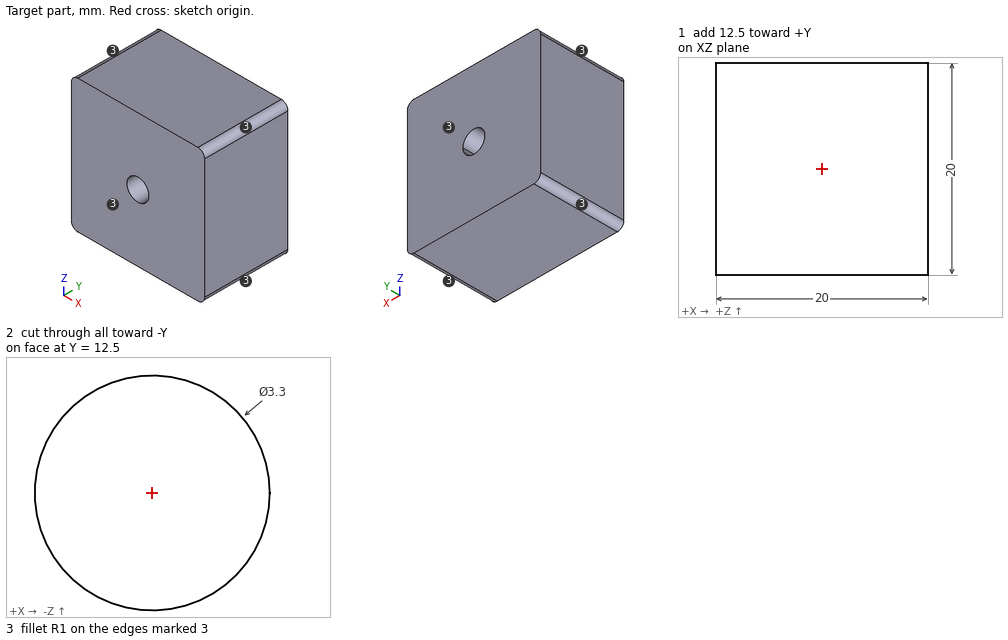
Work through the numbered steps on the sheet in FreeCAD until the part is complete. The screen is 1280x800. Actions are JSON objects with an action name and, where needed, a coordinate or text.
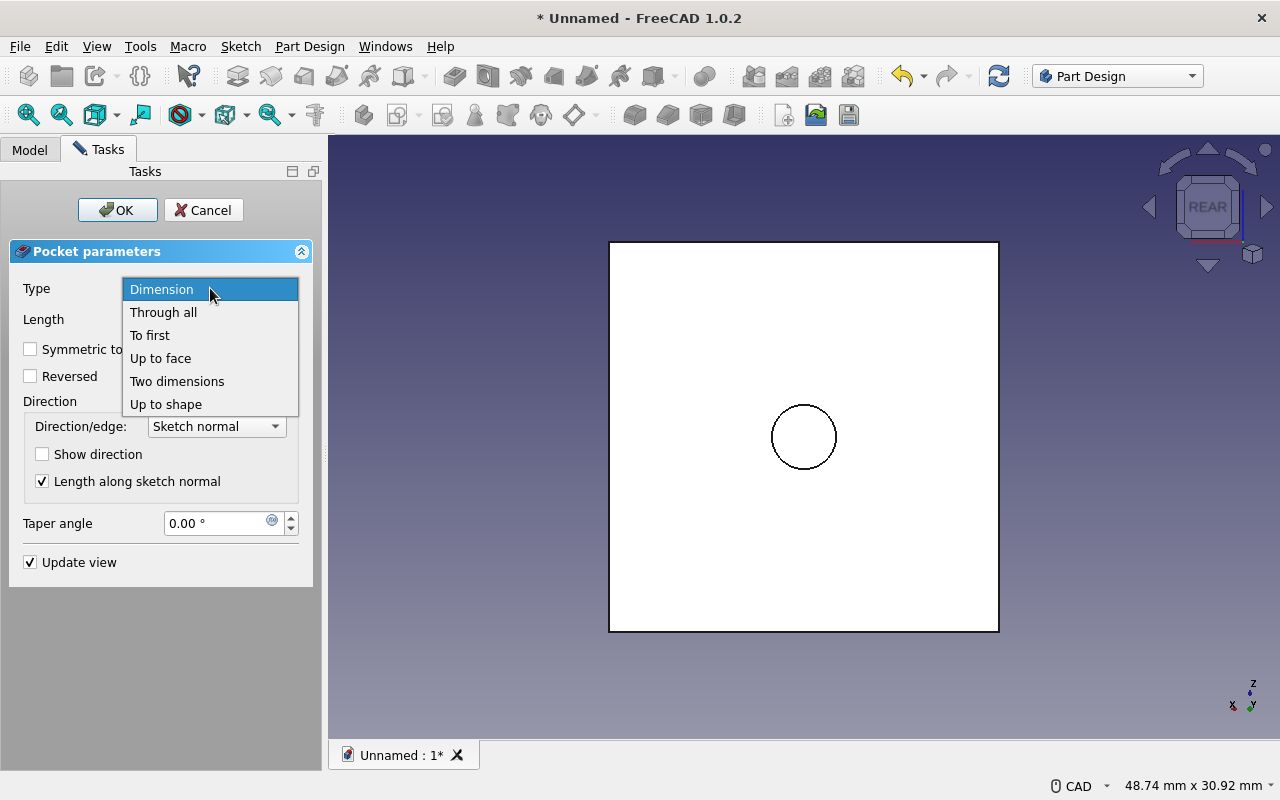
{"action": "left_click", "coordinate": [208, 312]}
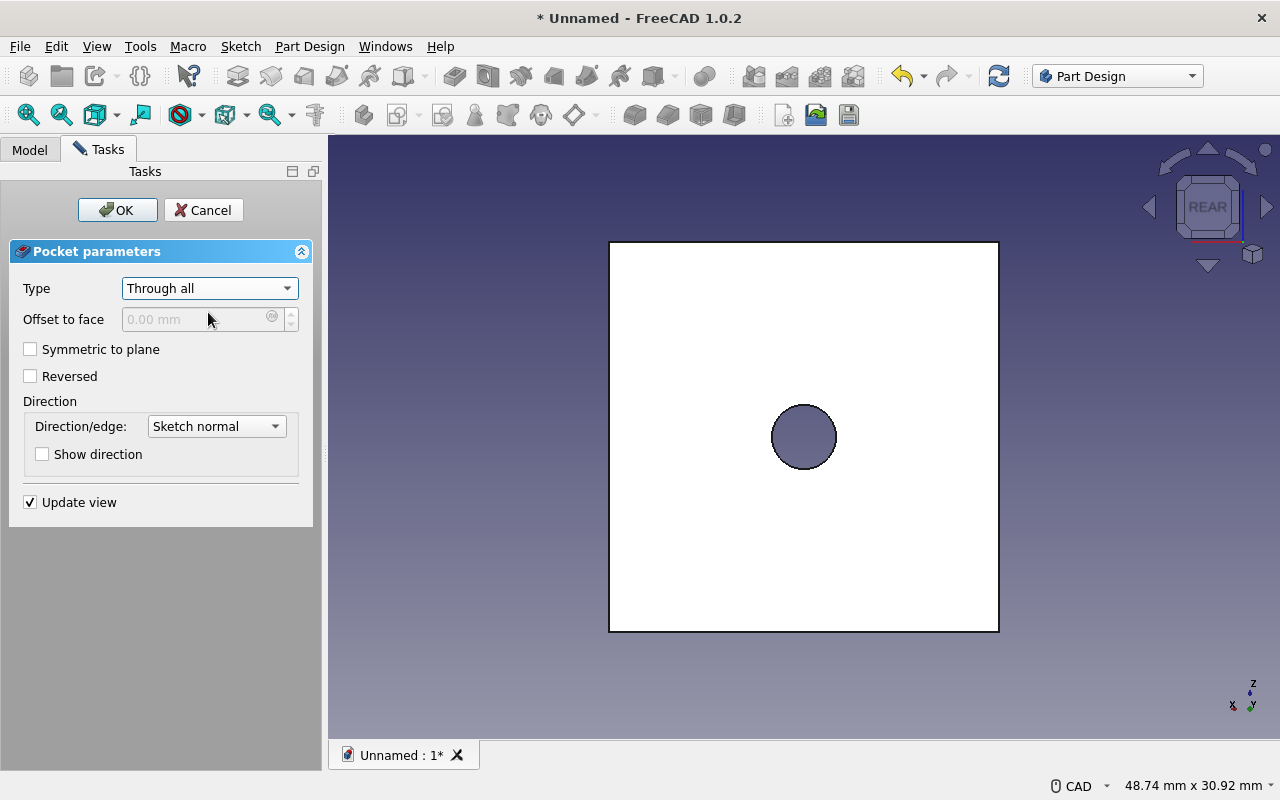
{"action": "left_click", "coordinate": [118, 210]}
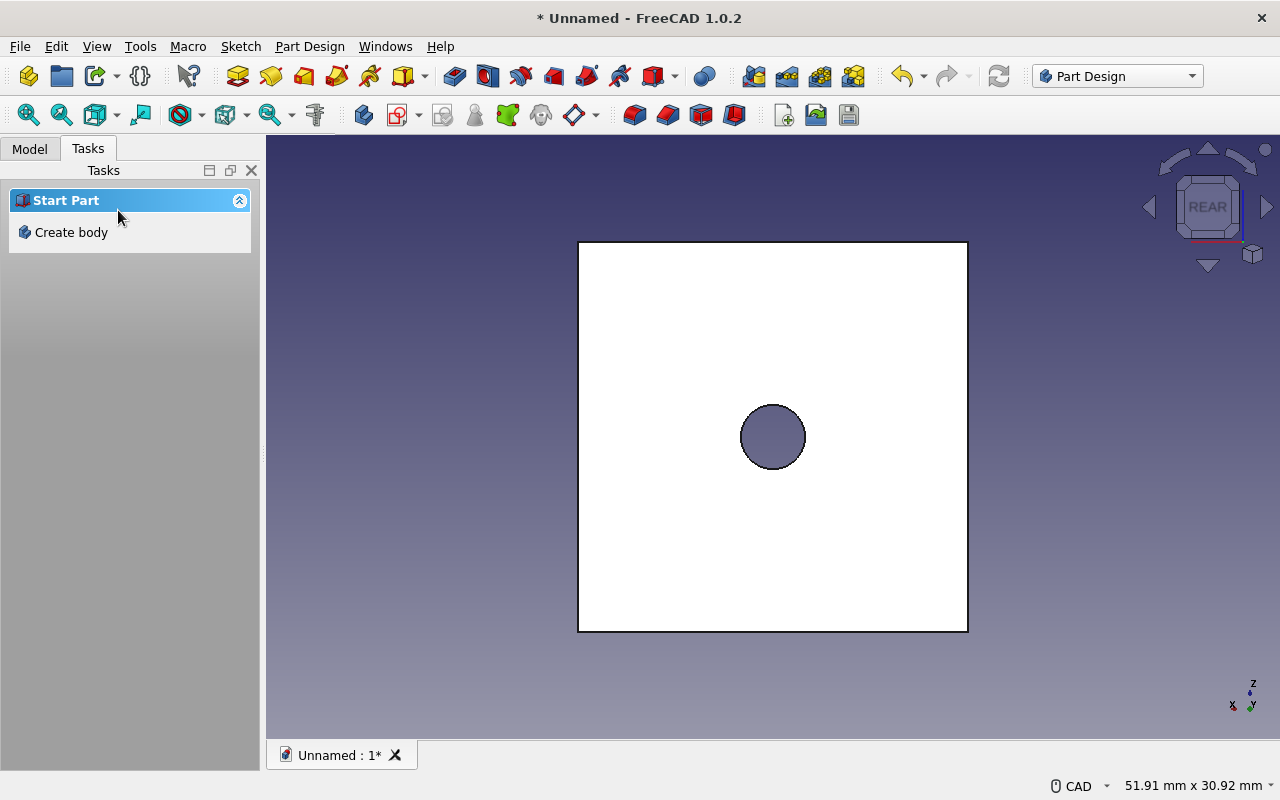
{"action": "key", "text": "0"}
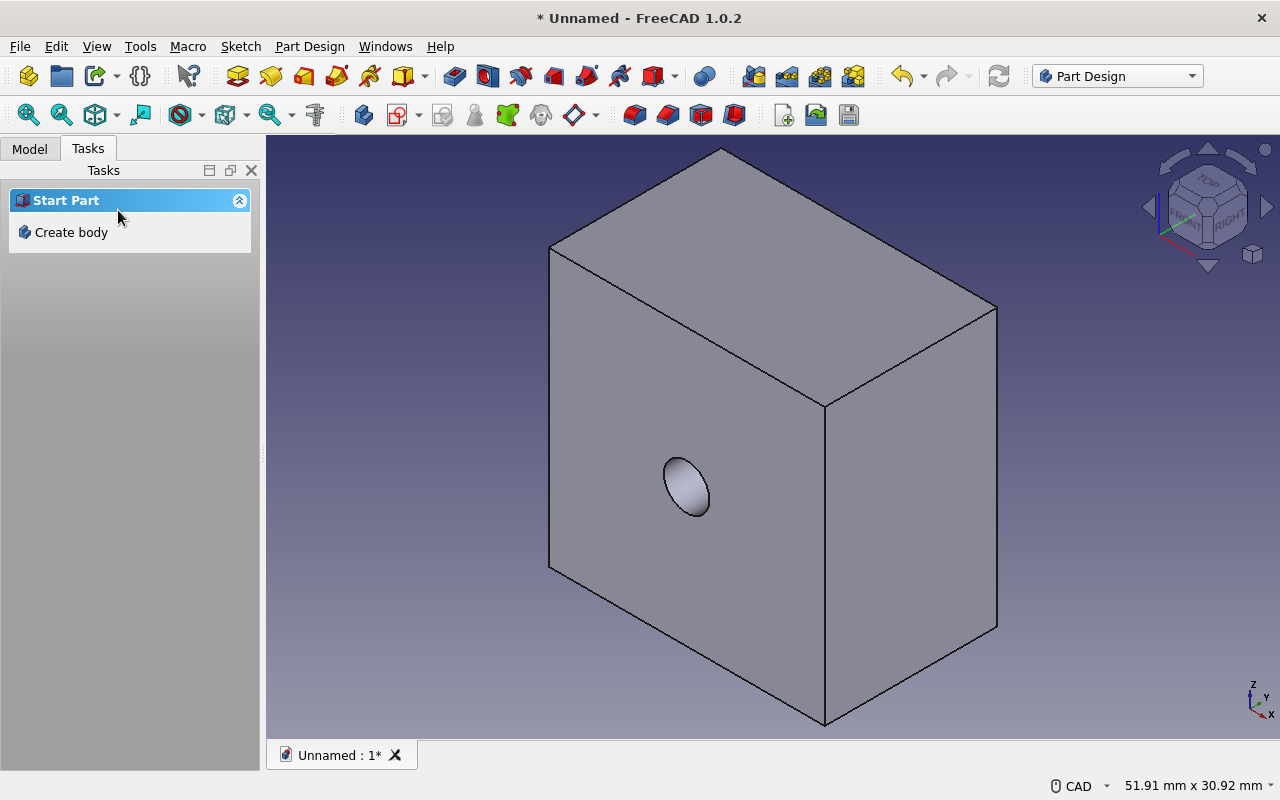
{"action": "left_click", "coordinate": [911, 356]}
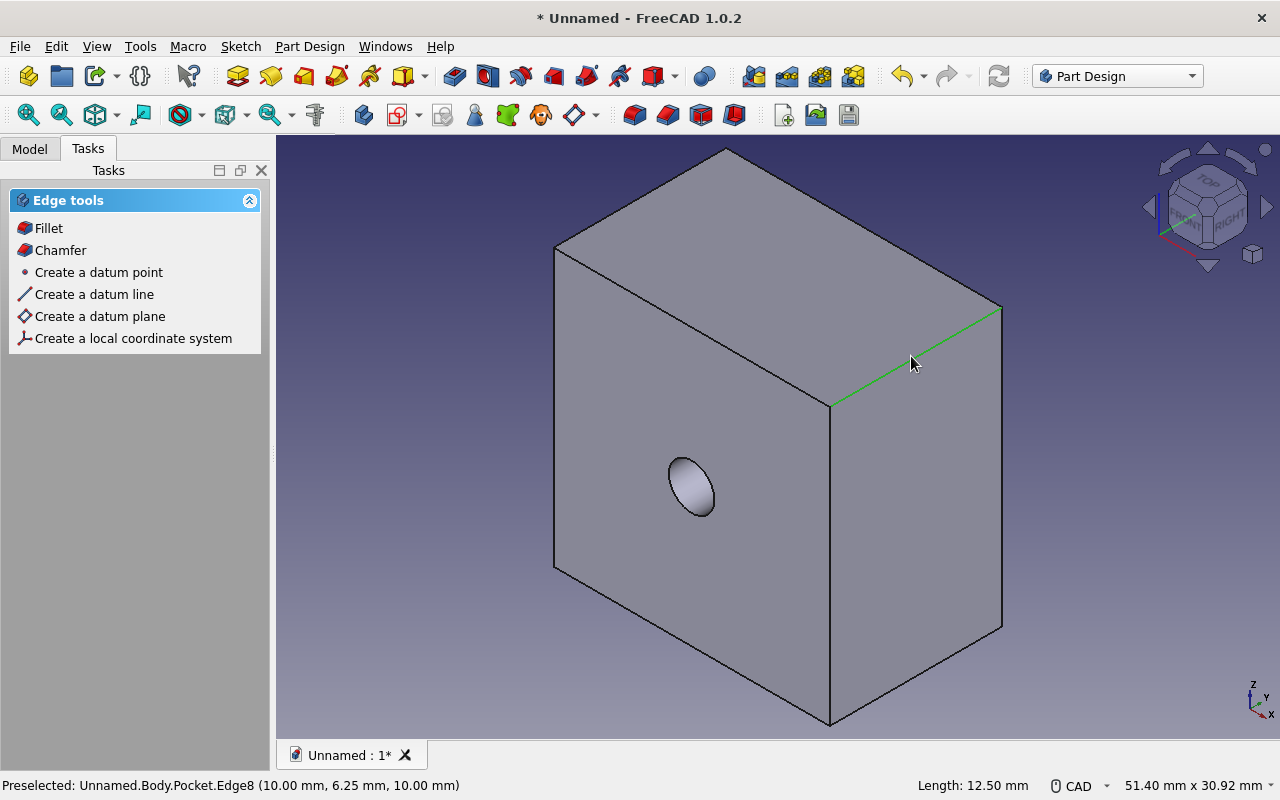
{"action": "key", "text": "2"}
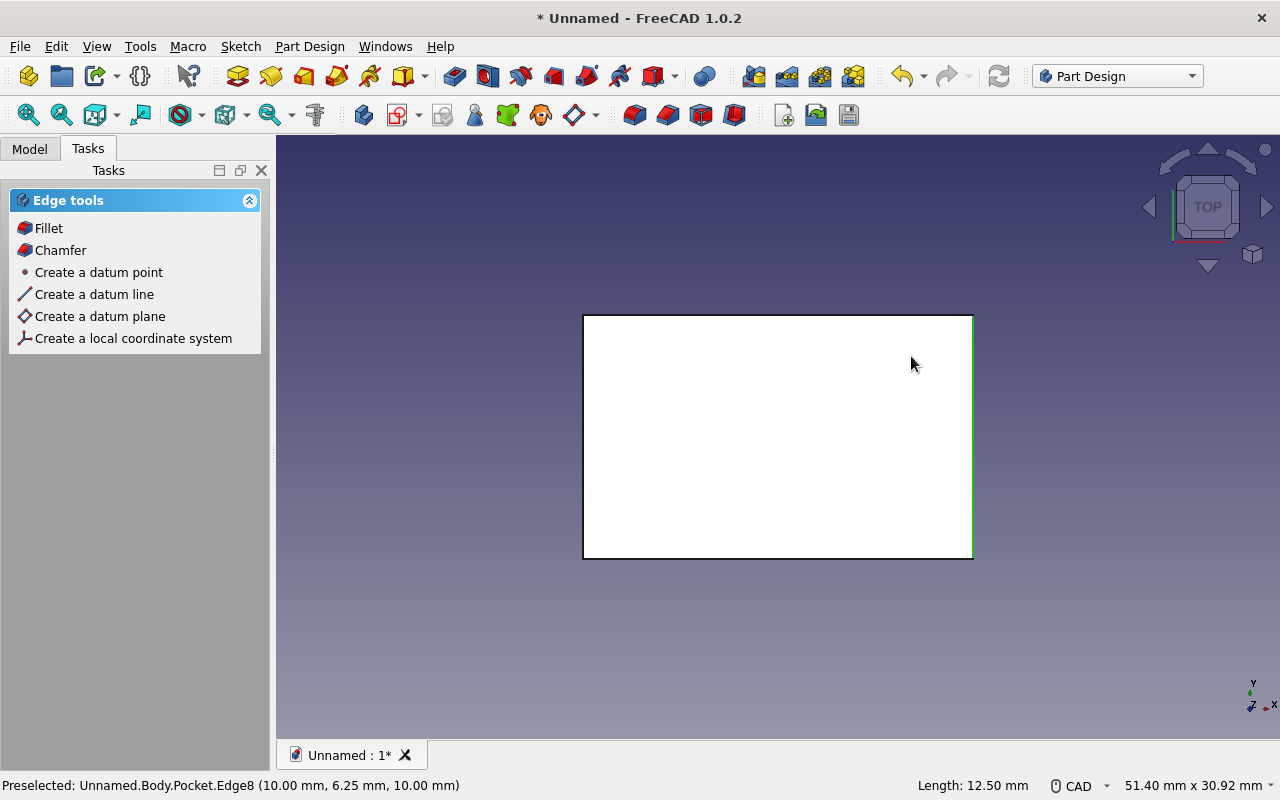
{"action": "left_click", "coordinate": [29, 116]}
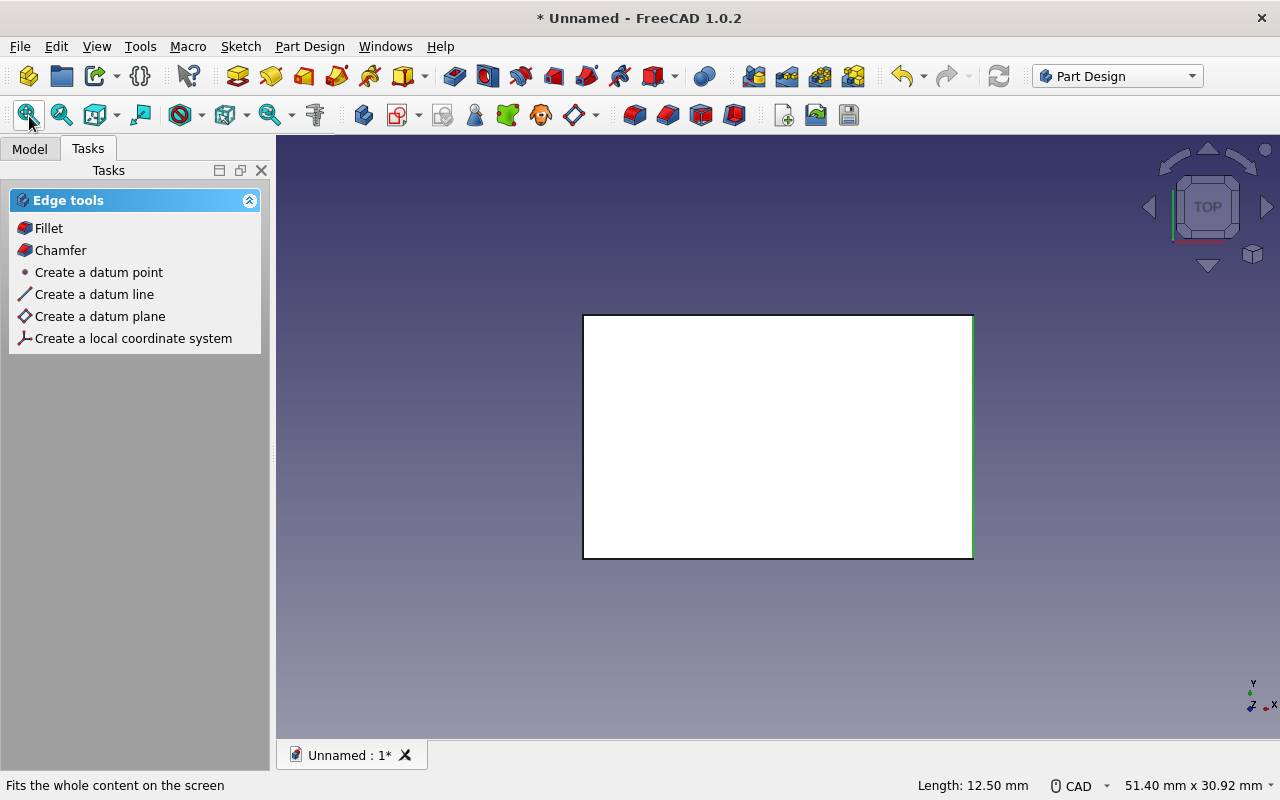
{"action": "left_click", "coordinate": [583, 436], "text": "ctrl"}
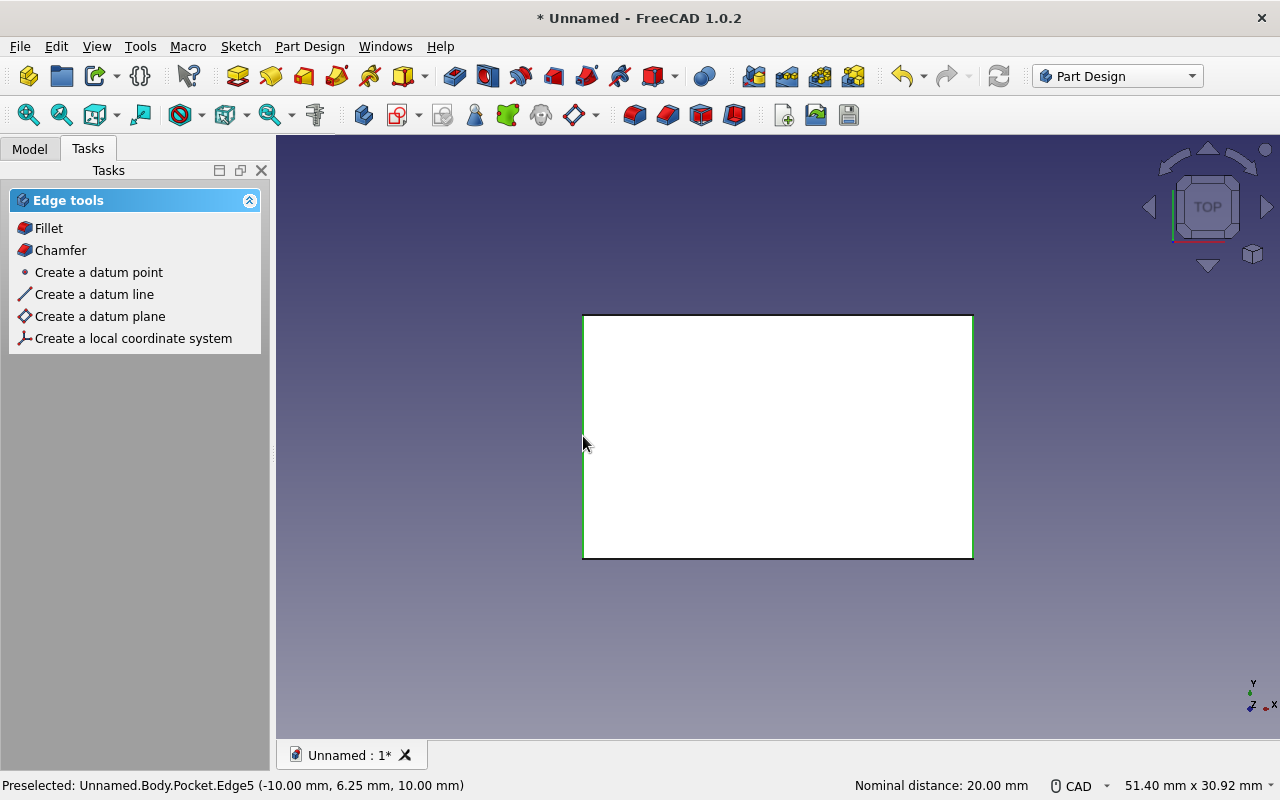
{"action": "key", "text": "1"}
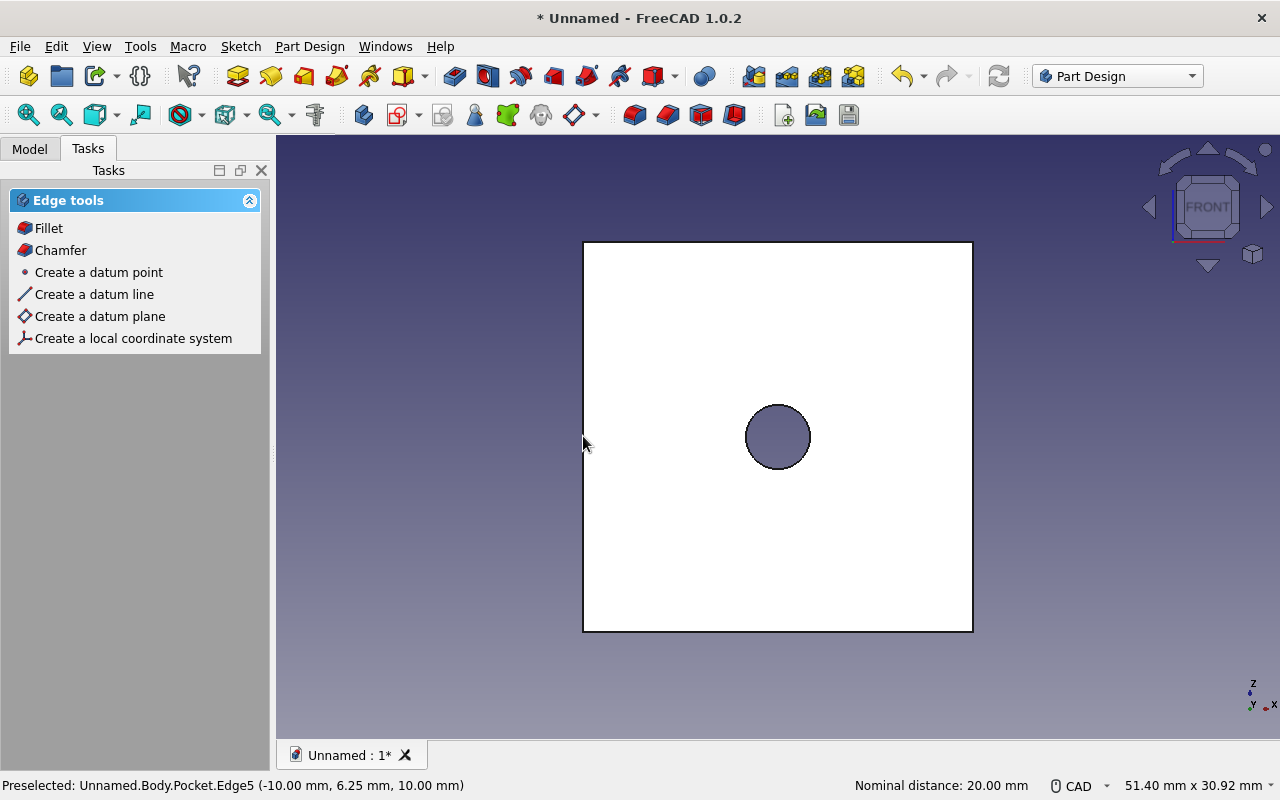
{"action": "key", "text": "3"}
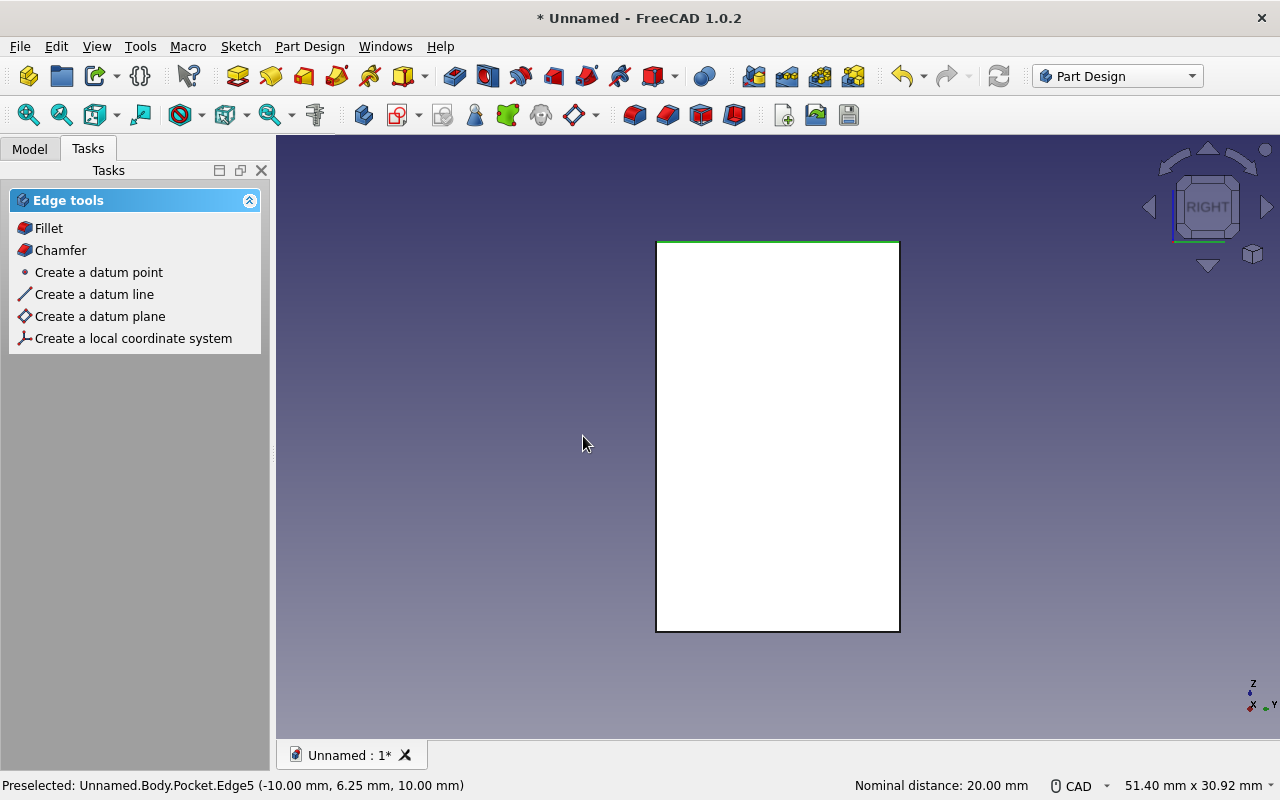
{"action": "left_click", "coordinate": [778, 631], "text": "ctrl"}